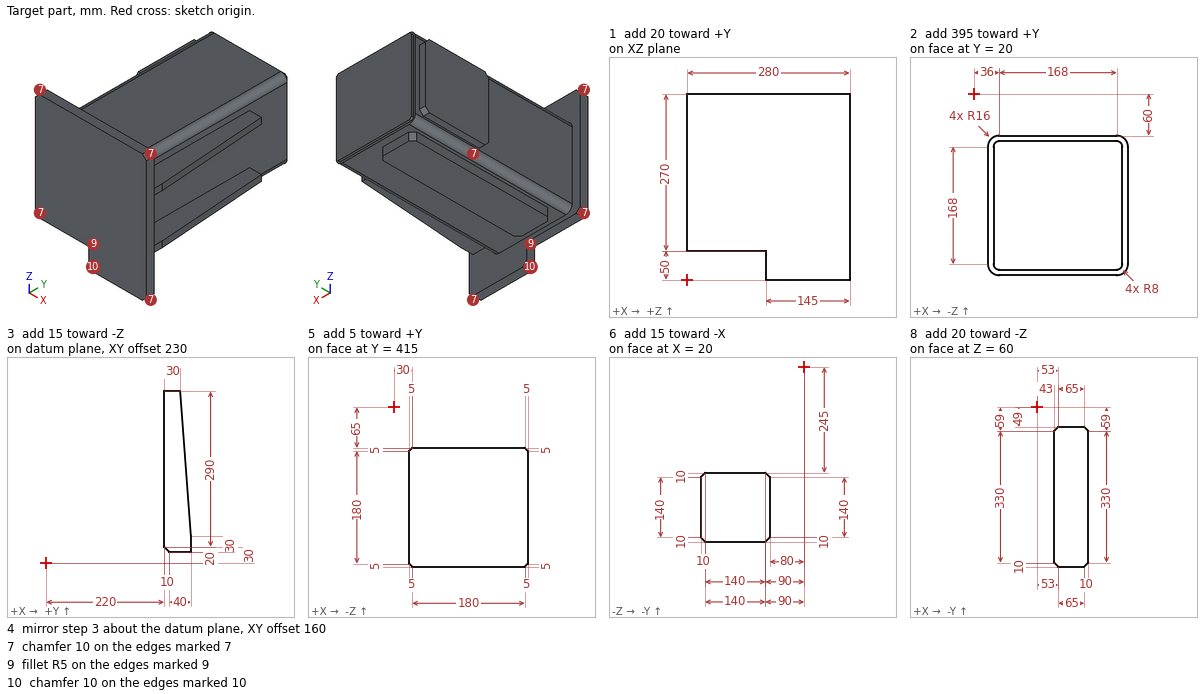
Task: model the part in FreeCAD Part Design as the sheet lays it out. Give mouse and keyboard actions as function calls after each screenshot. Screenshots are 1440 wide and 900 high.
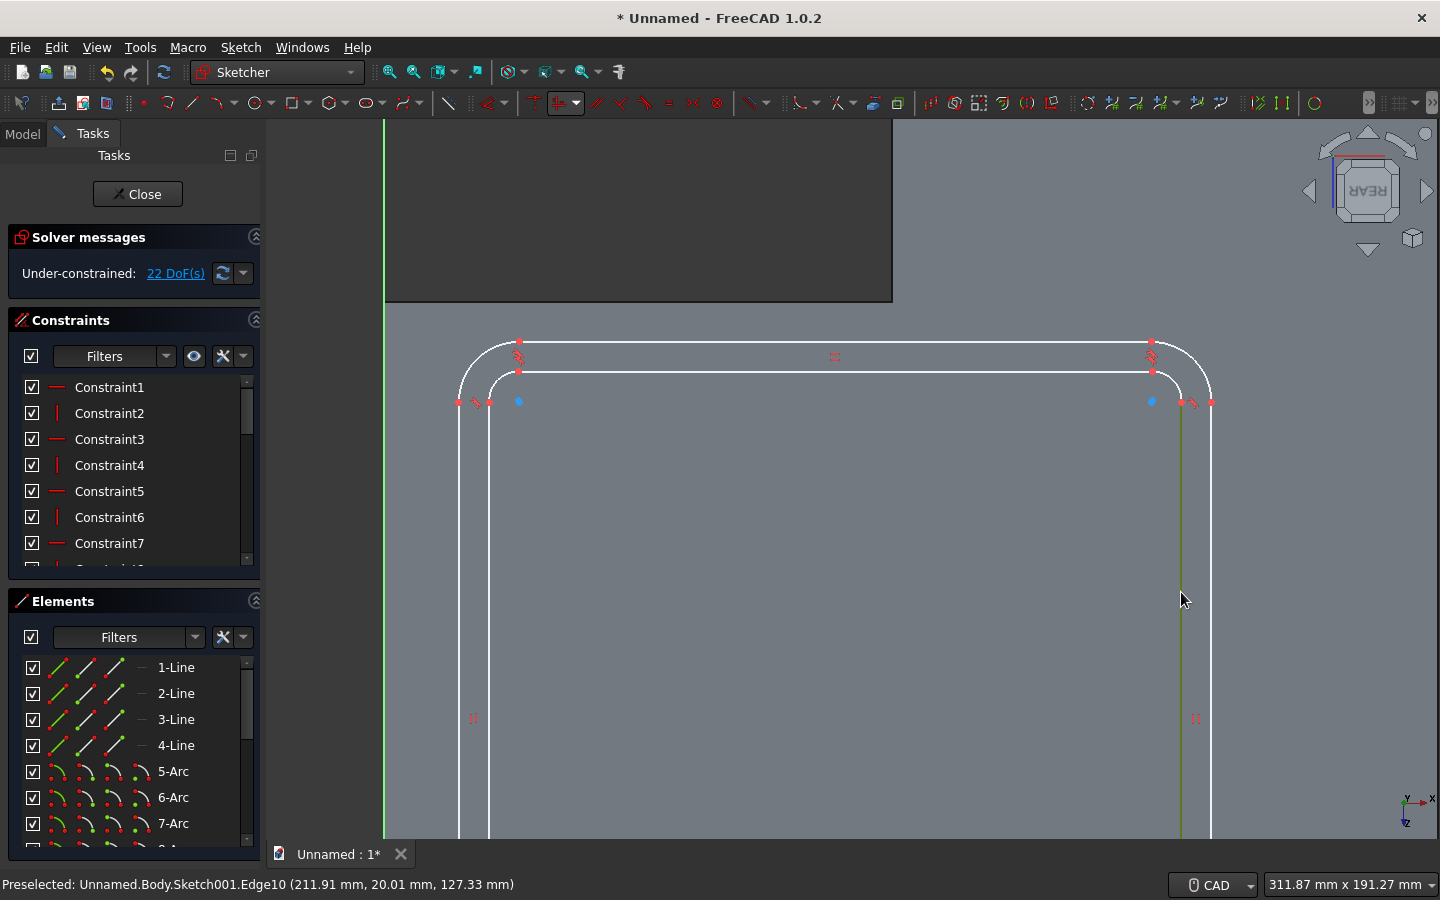
click(1179, 389)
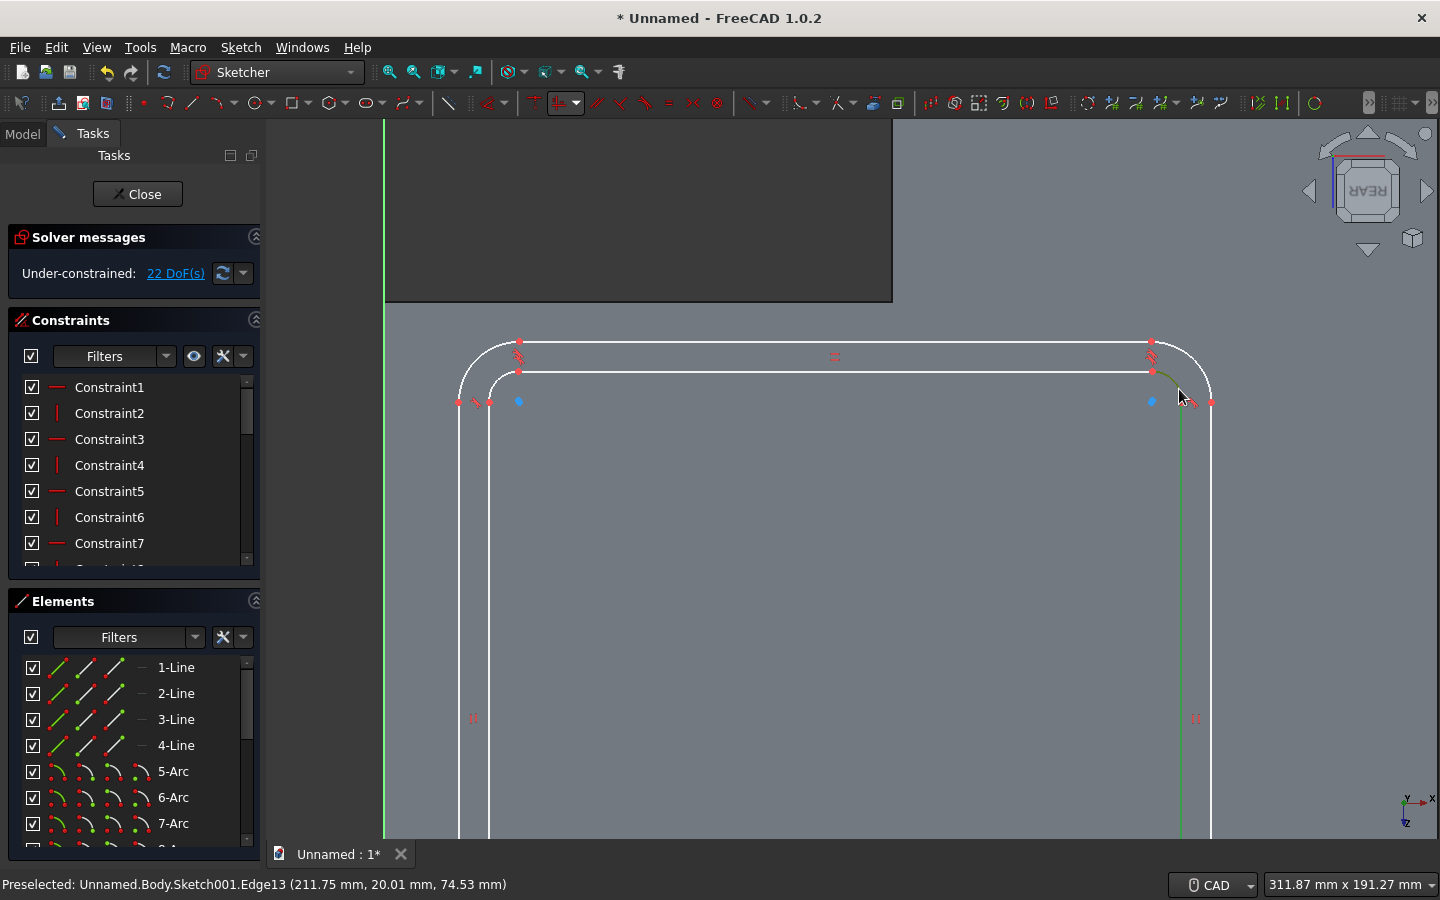
click(646, 104)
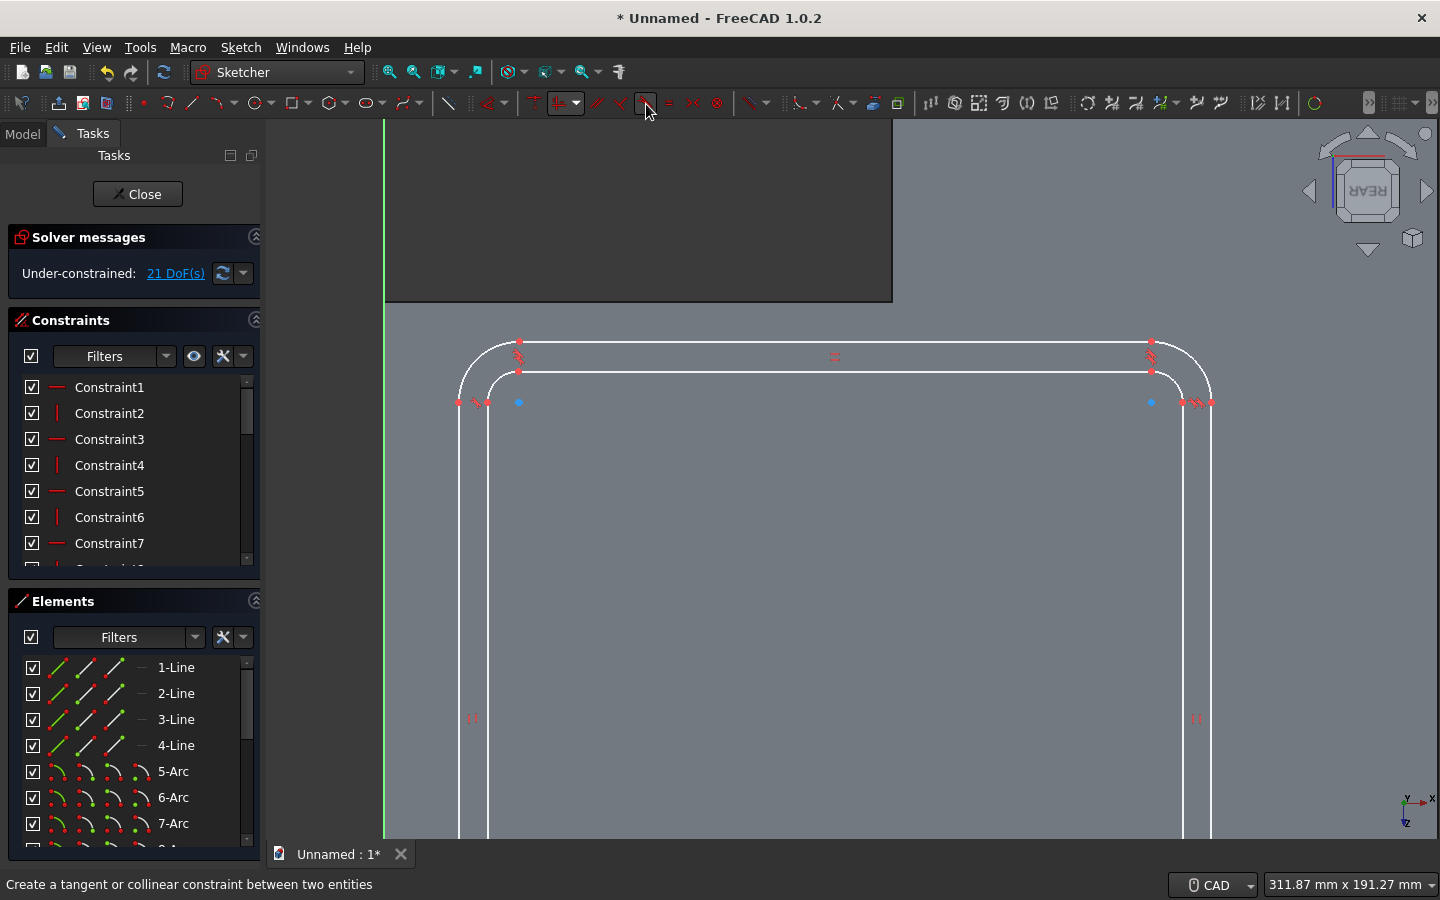
click(1183, 592)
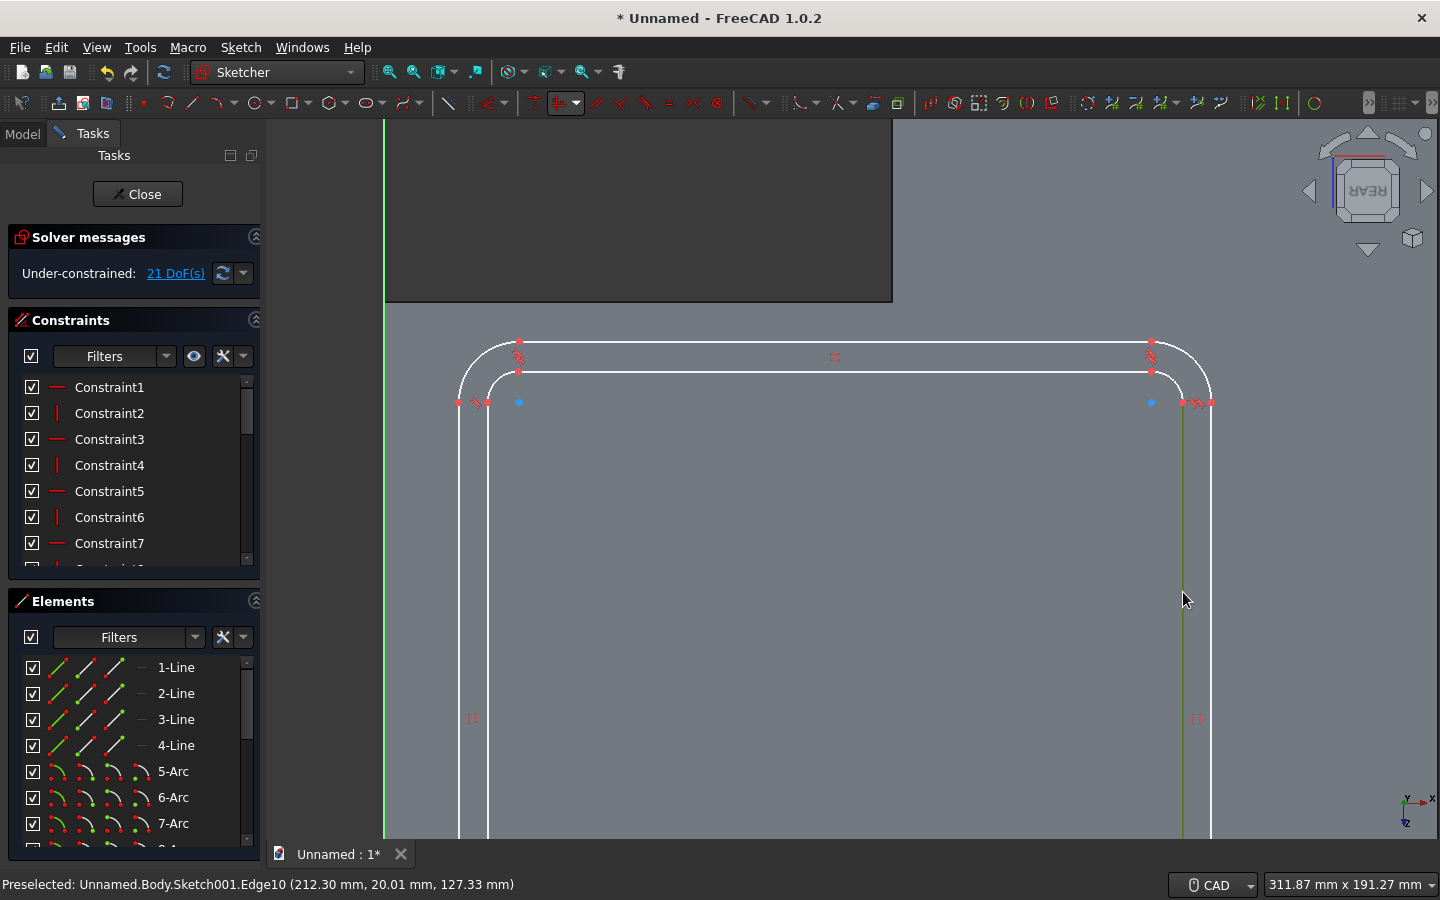
scroll(774, 378, down, 4)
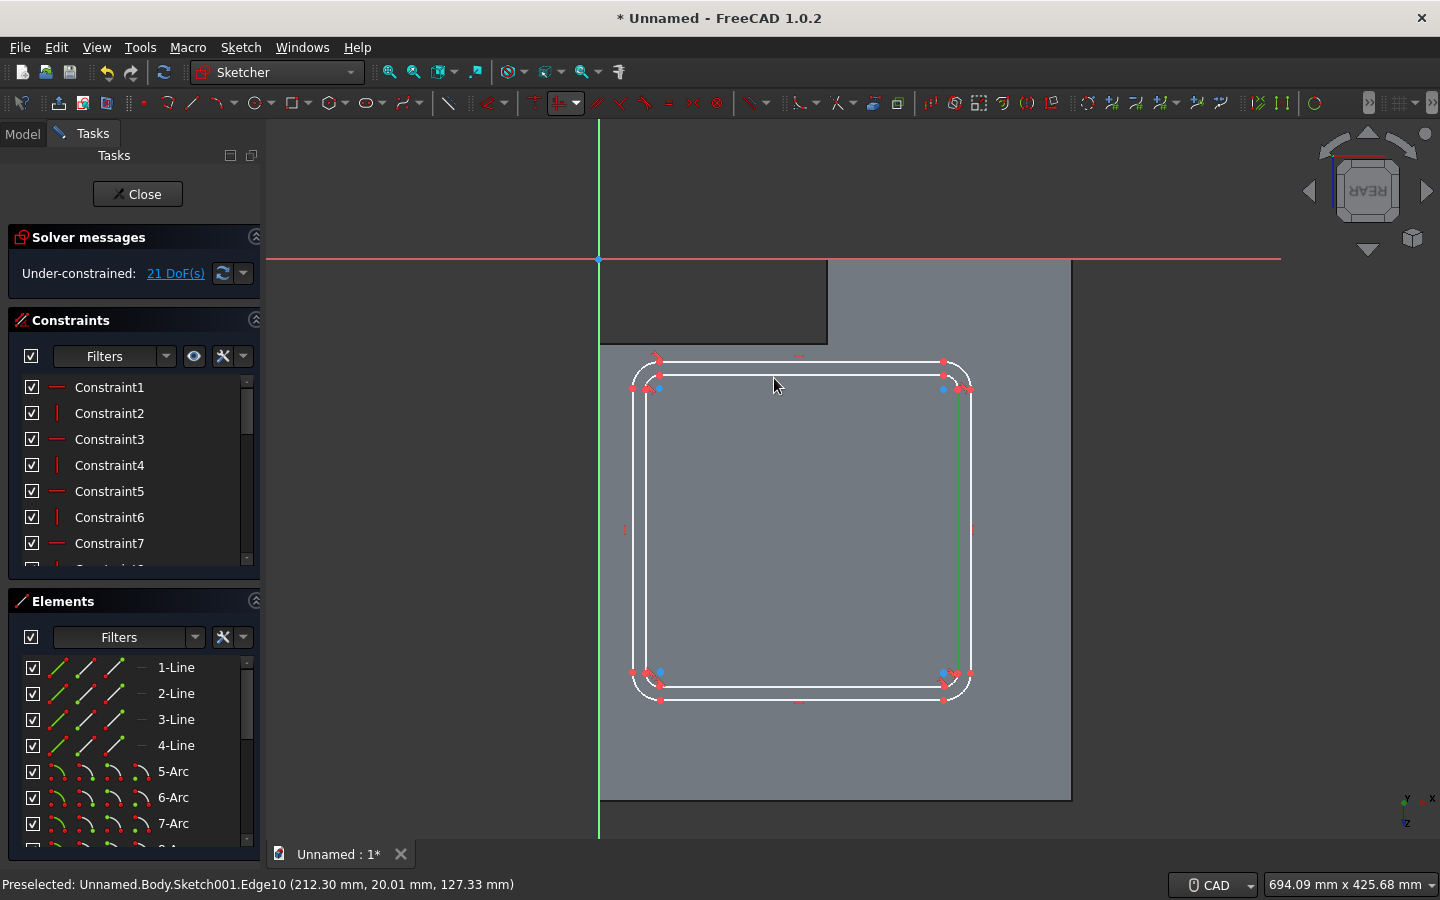
scroll(950, 685, up, 4)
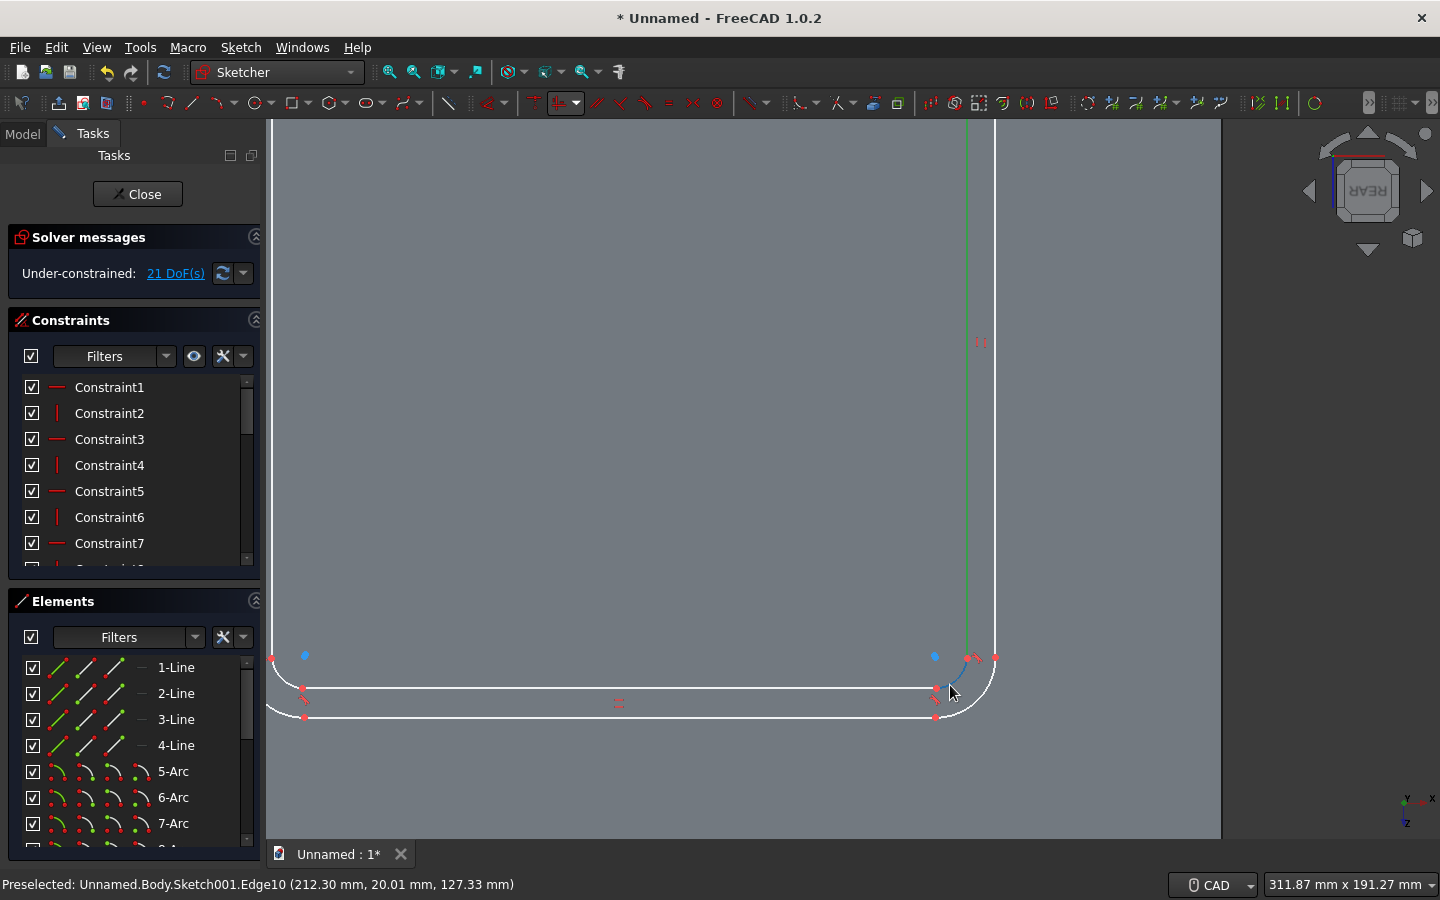
click(950, 684)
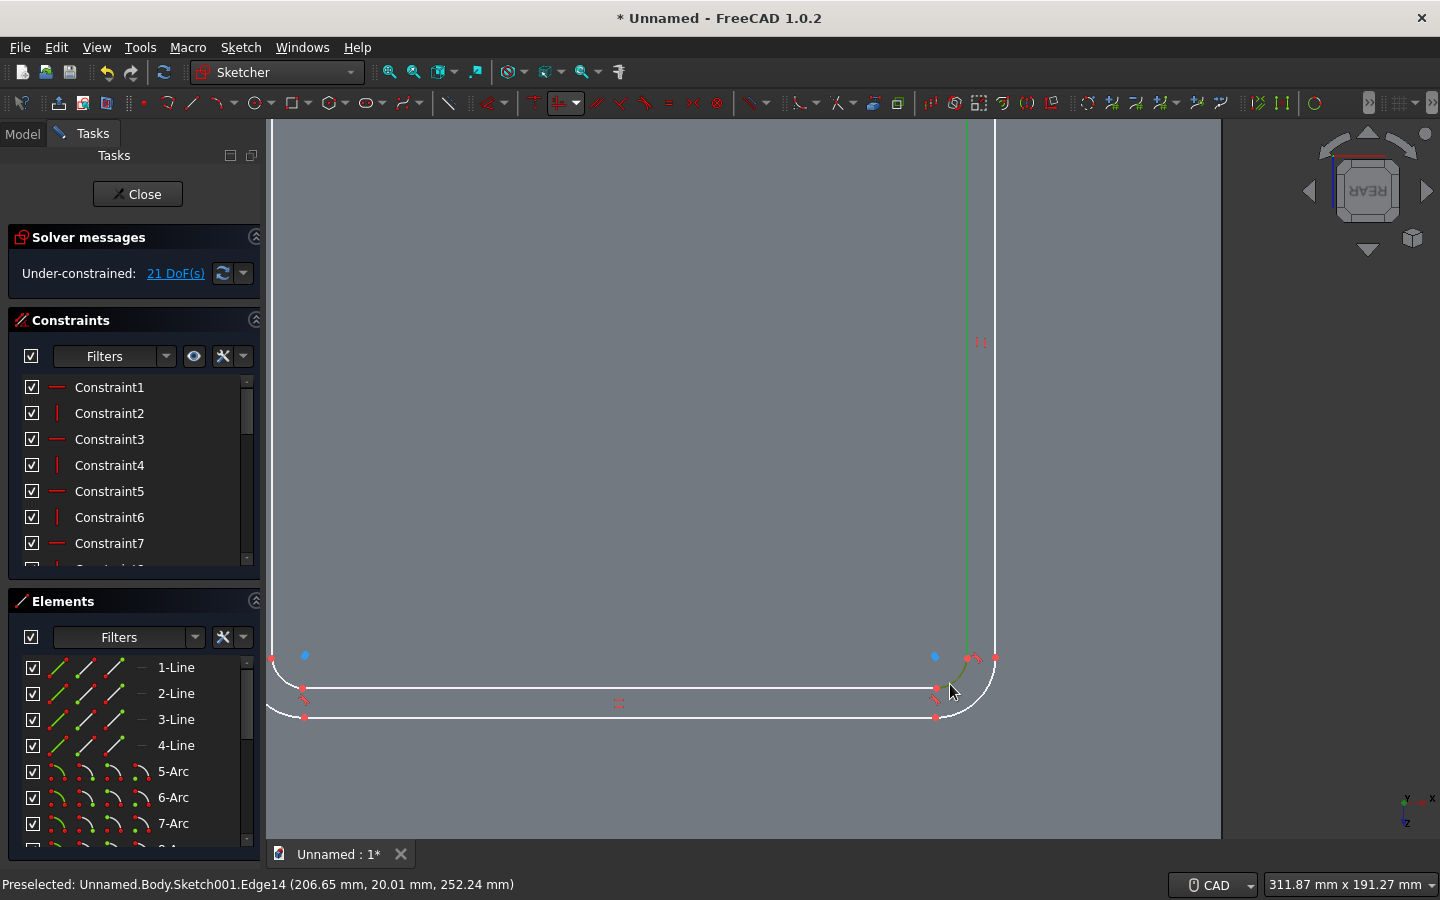
click(646, 104)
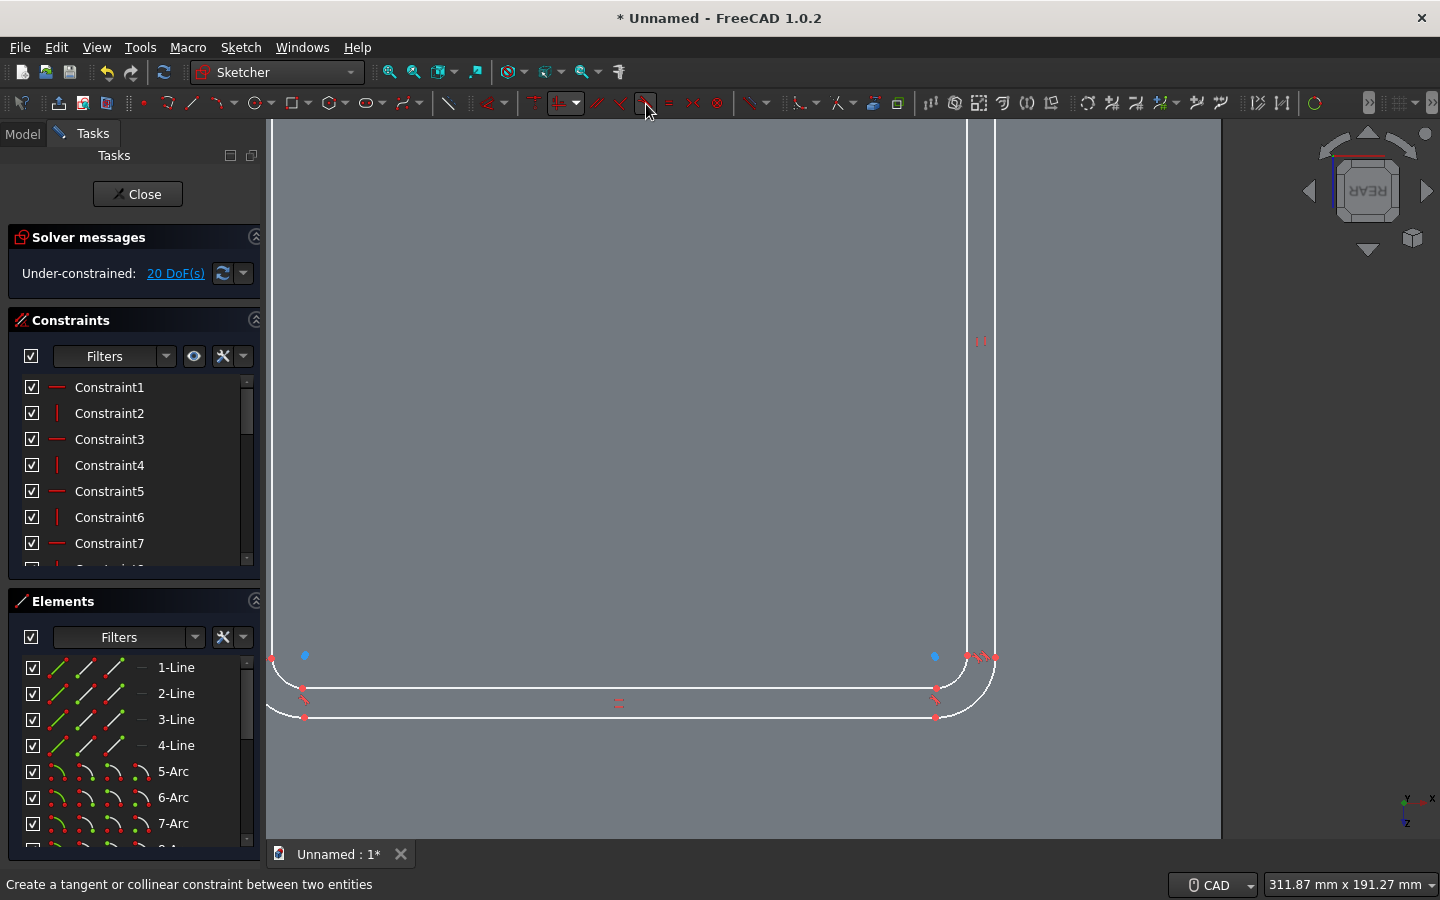
click(746, 688)